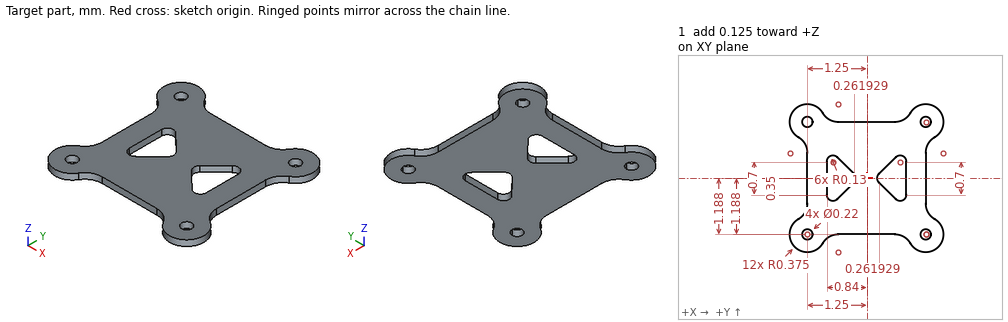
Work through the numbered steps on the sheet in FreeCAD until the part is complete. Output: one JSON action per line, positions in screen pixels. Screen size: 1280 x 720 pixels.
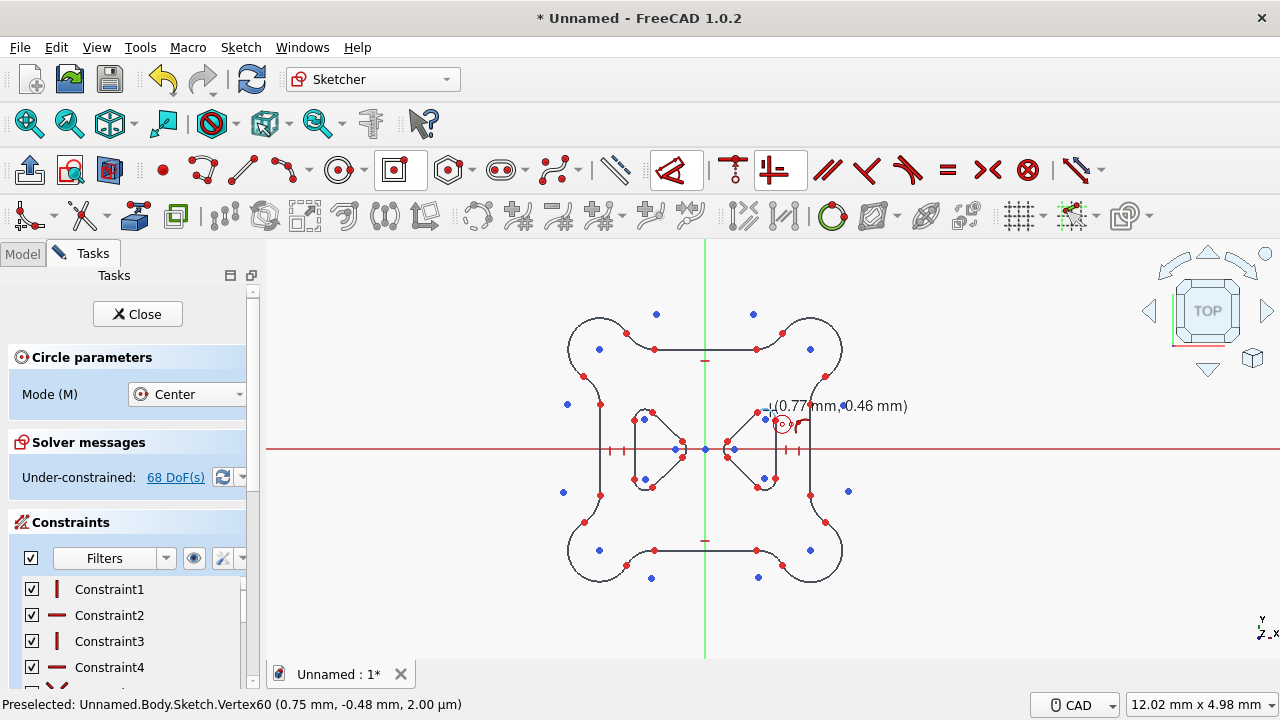
{"action": "scroll", "coordinate": [600, 549], "scroll_direction": "up", "scroll_amount": 5}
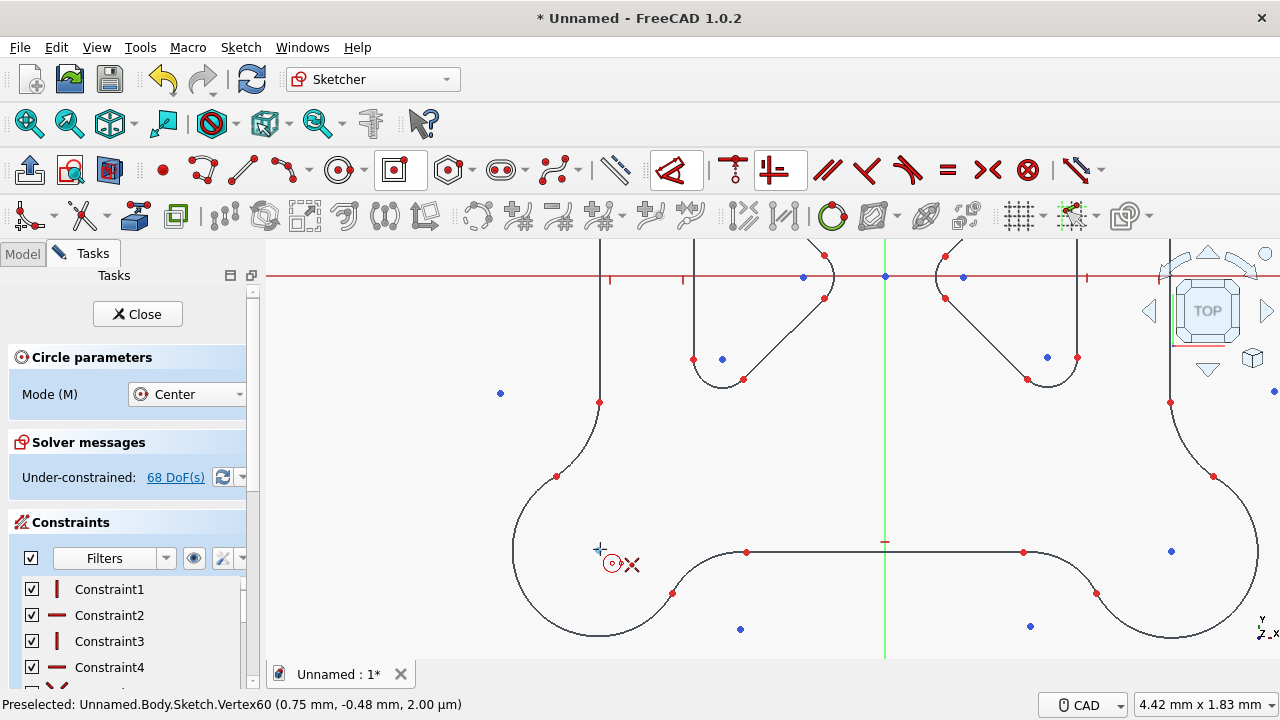
{"action": "left_click", "coordinate": [598, 549]}
{"action": "left_click", "coordinate": [616, 531]}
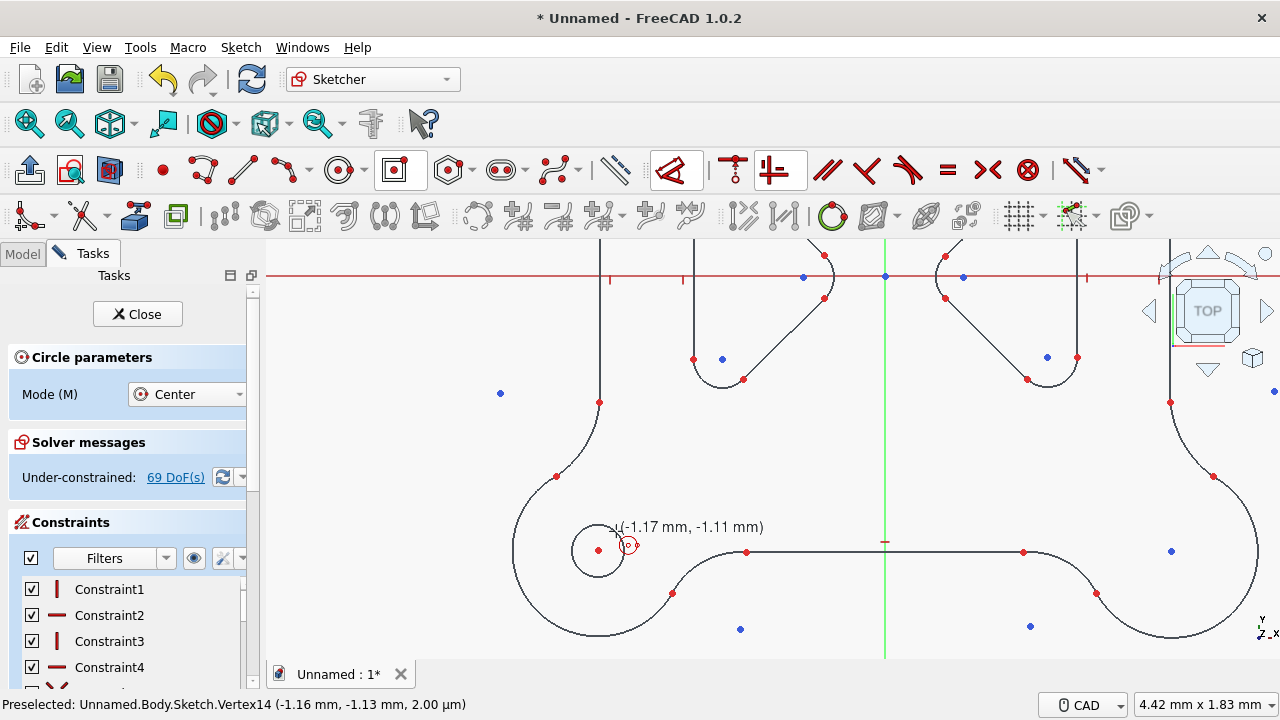
{"action": "scroll", "coordinate": [599, 549], "scroll_direction": "down", "scroll_amount": 5}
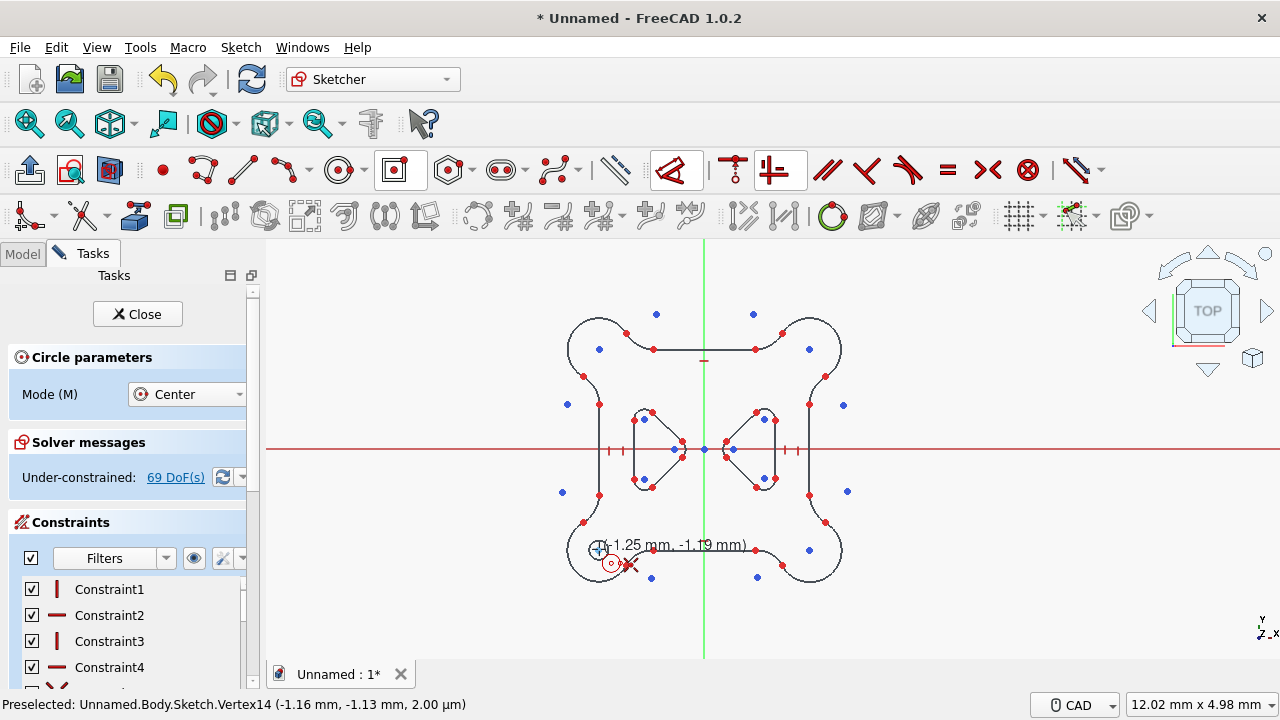
{"action": "scroll", "coordinate": [810, 549], "scroll_direction": "up", "scroll_amount": 5}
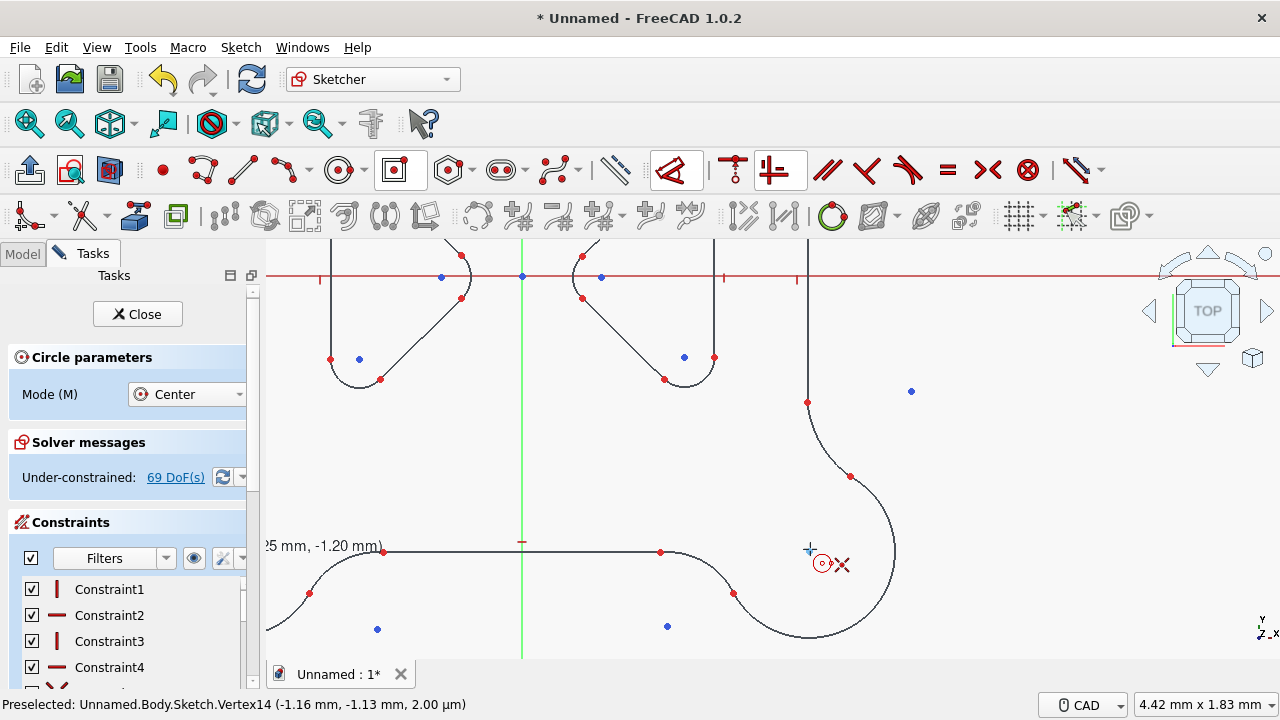
{"action": "left_click", "coordinate": [809, 549]}
{"action": "left_click", "coordinate": [827, 531]}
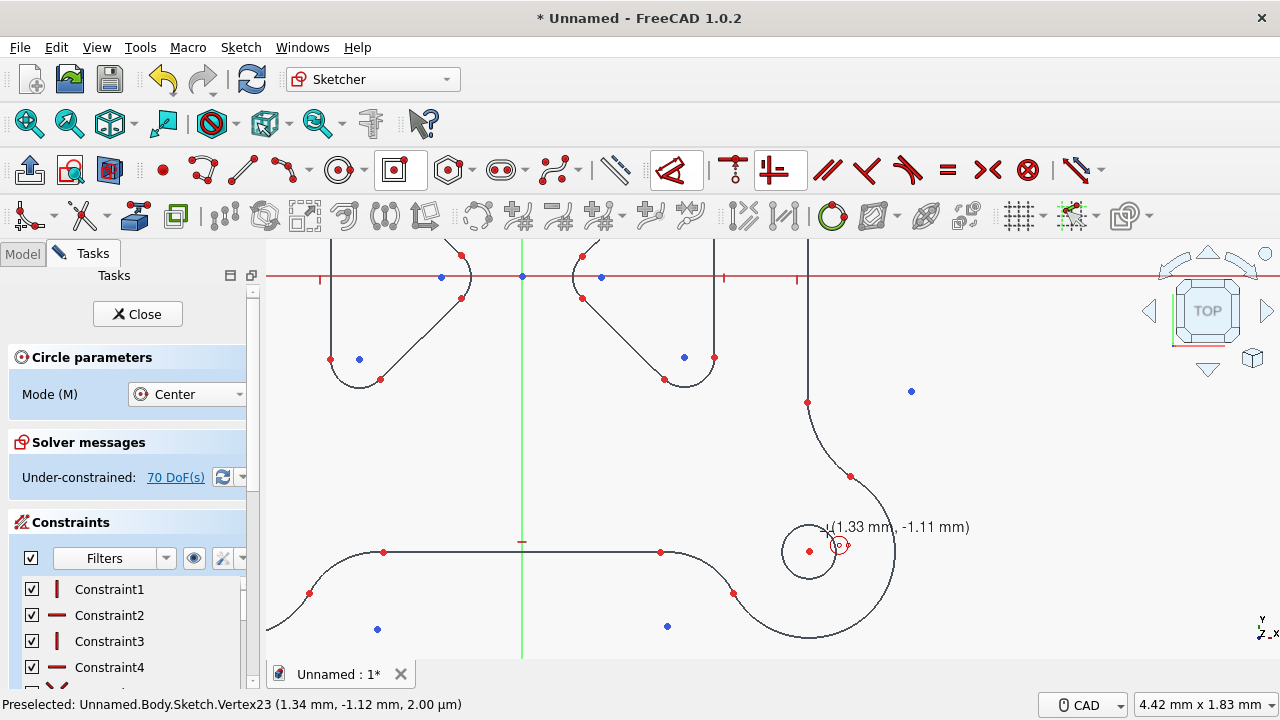
{"action": "scroll", "coordinate": [811, 549], "scroll_direction": "down", "scroll_amount": 5}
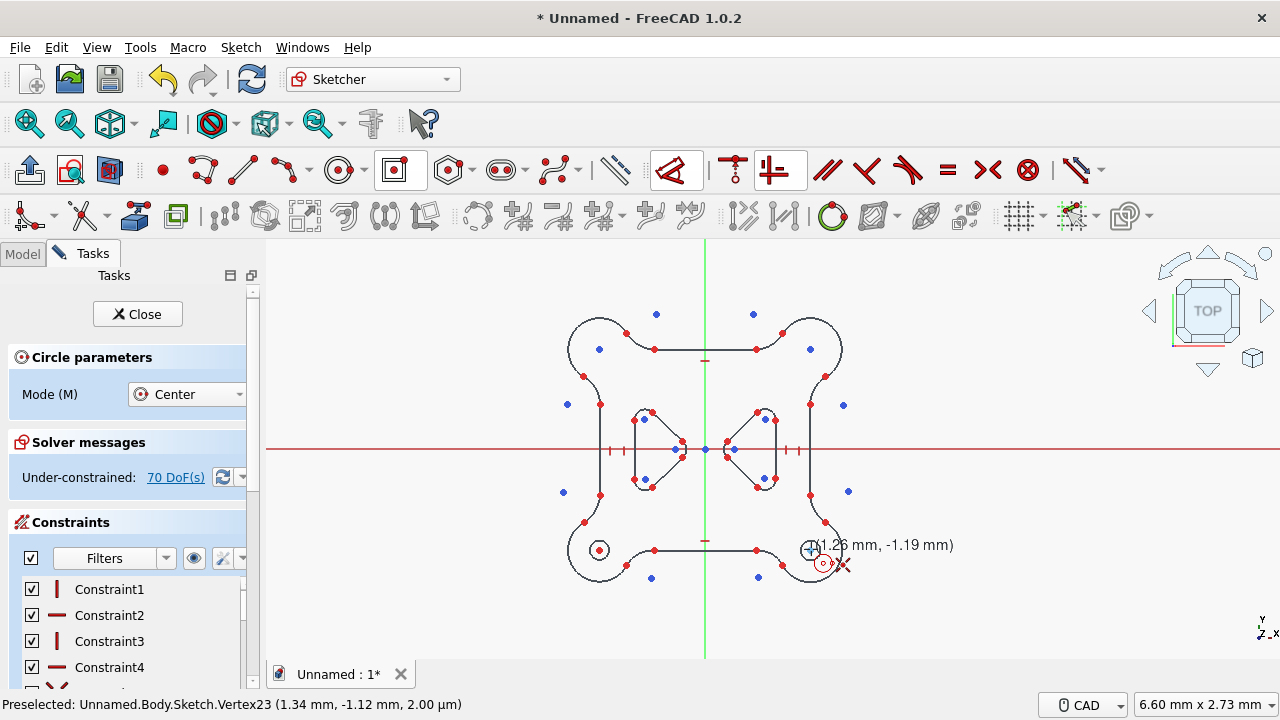
{"action": "scroll", "coordinate": [600, 349], "scroll_direction": "up", "scroll_amount": 5}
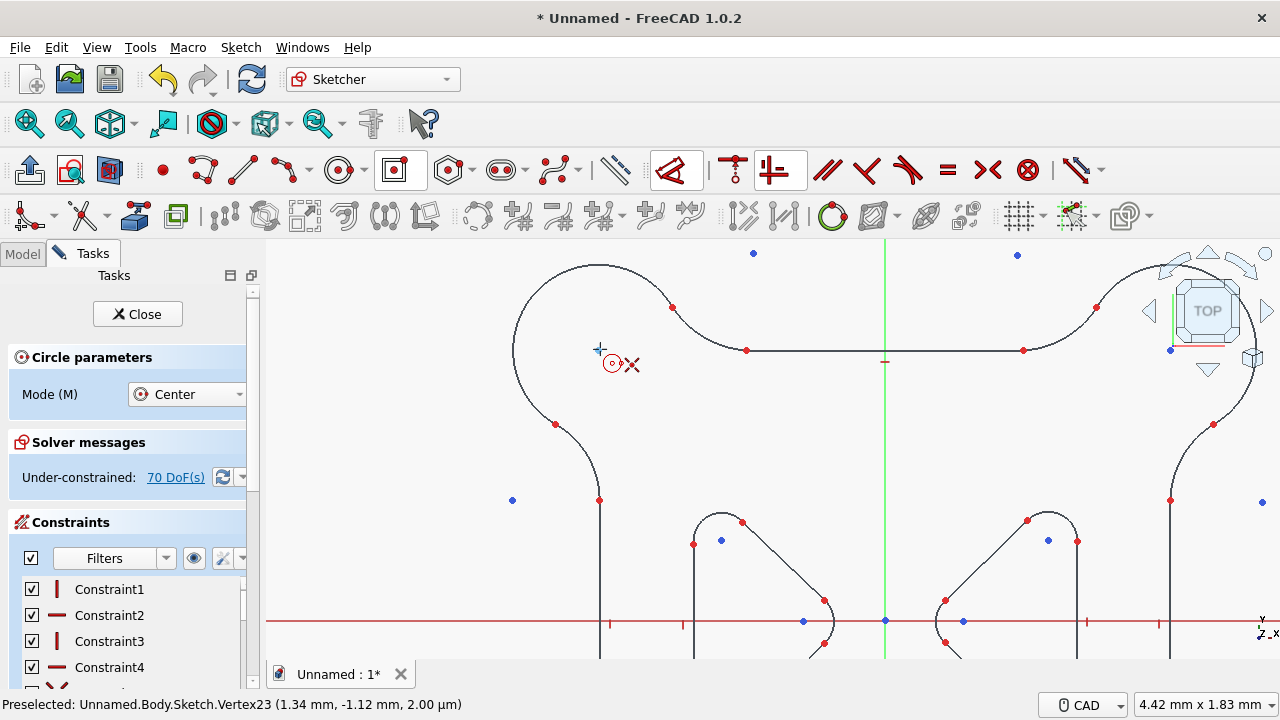
{"action": "left_click", "coordinate": [598, 348]}
{"action": "left_click", "coordinate": [616, 331]}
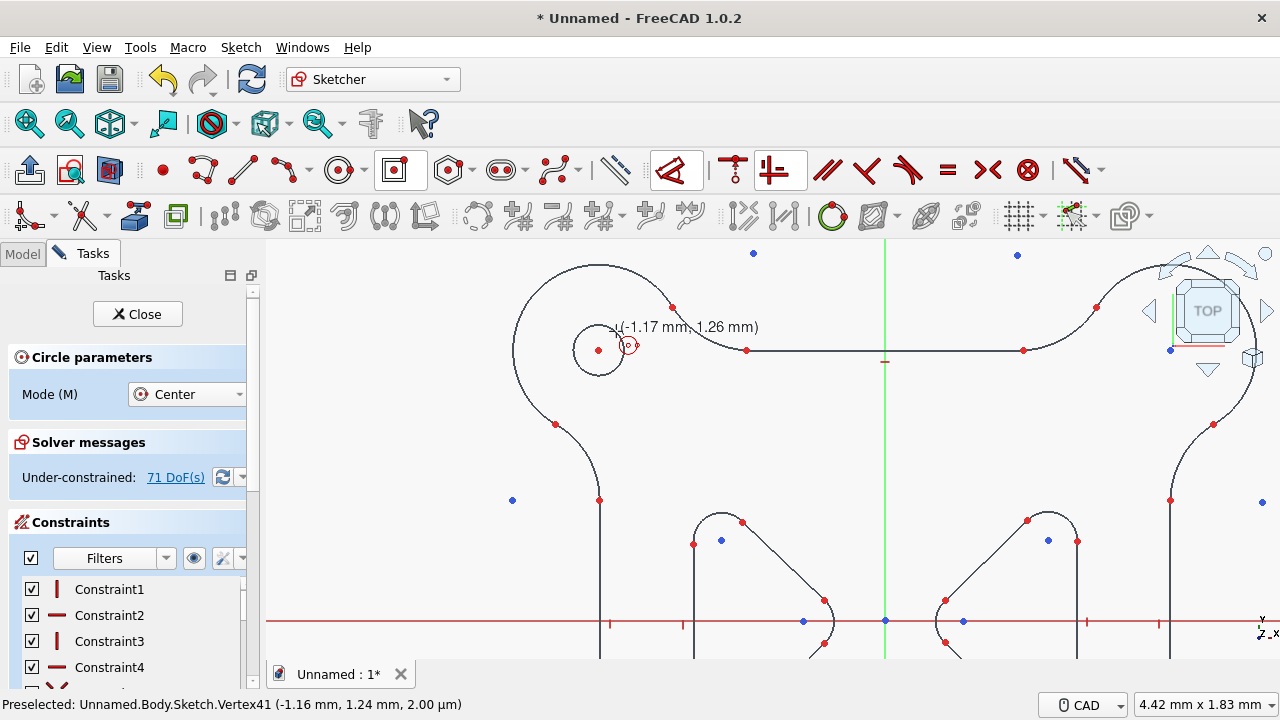
{"action": "scroll", "coordinate": [599, 349], "scroll_direction": "down", "scroll_amount": 5}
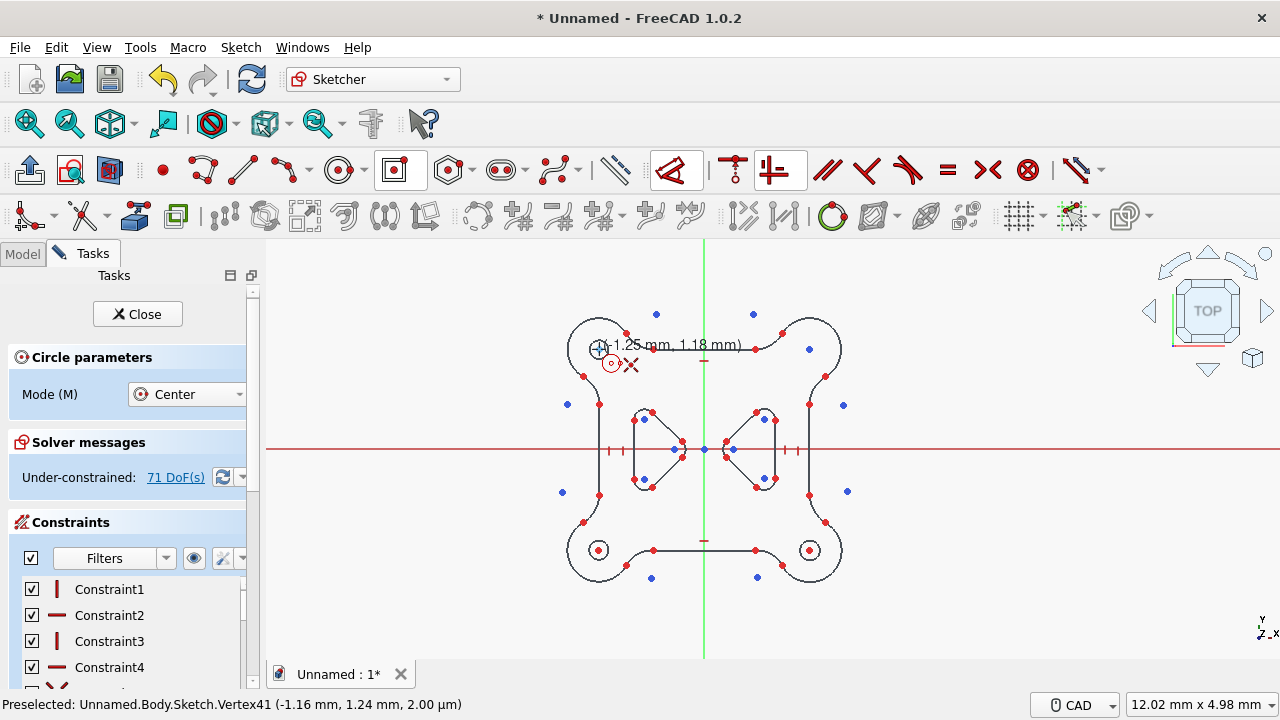
{"action": "scroll", "coordinate": [810, 349], "scroll_direction": "up", "scroll_amount": 5}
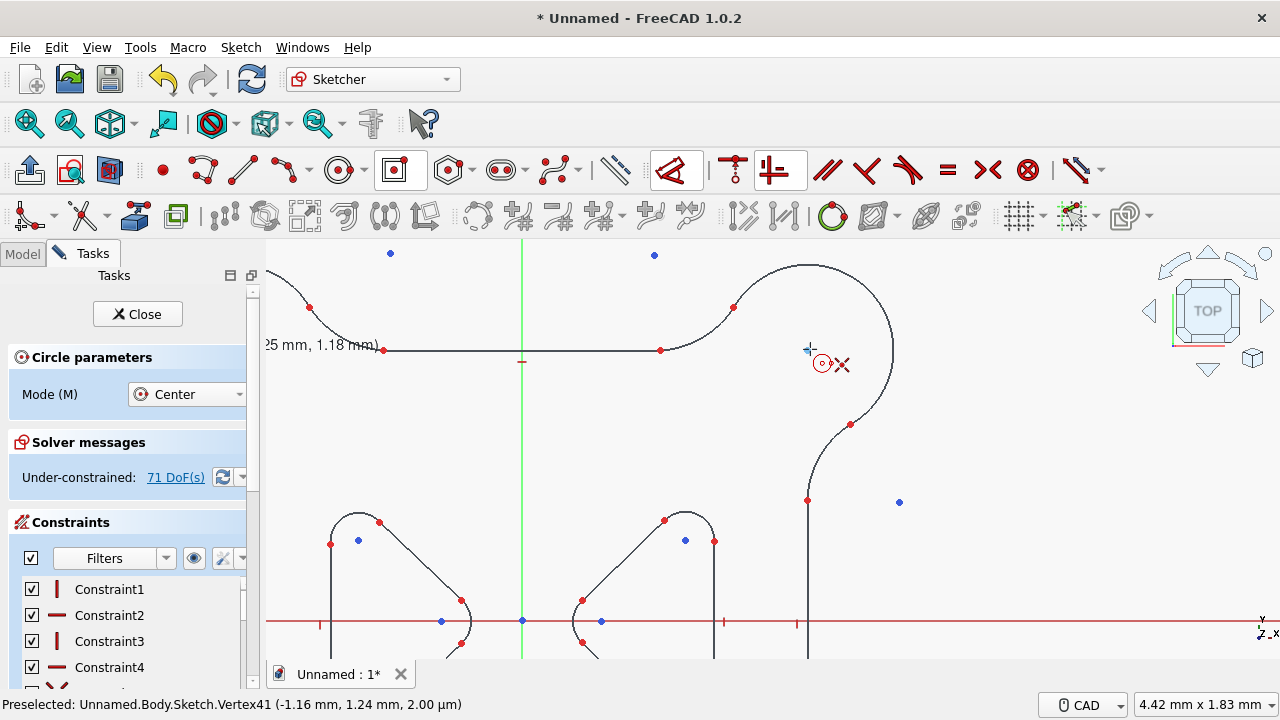
{"action": "left_click", "coordinate": [809, 348]}
{"action": "left_click", "coordinate": [827, 331]}
{"action": "key", "text": "Escape"}